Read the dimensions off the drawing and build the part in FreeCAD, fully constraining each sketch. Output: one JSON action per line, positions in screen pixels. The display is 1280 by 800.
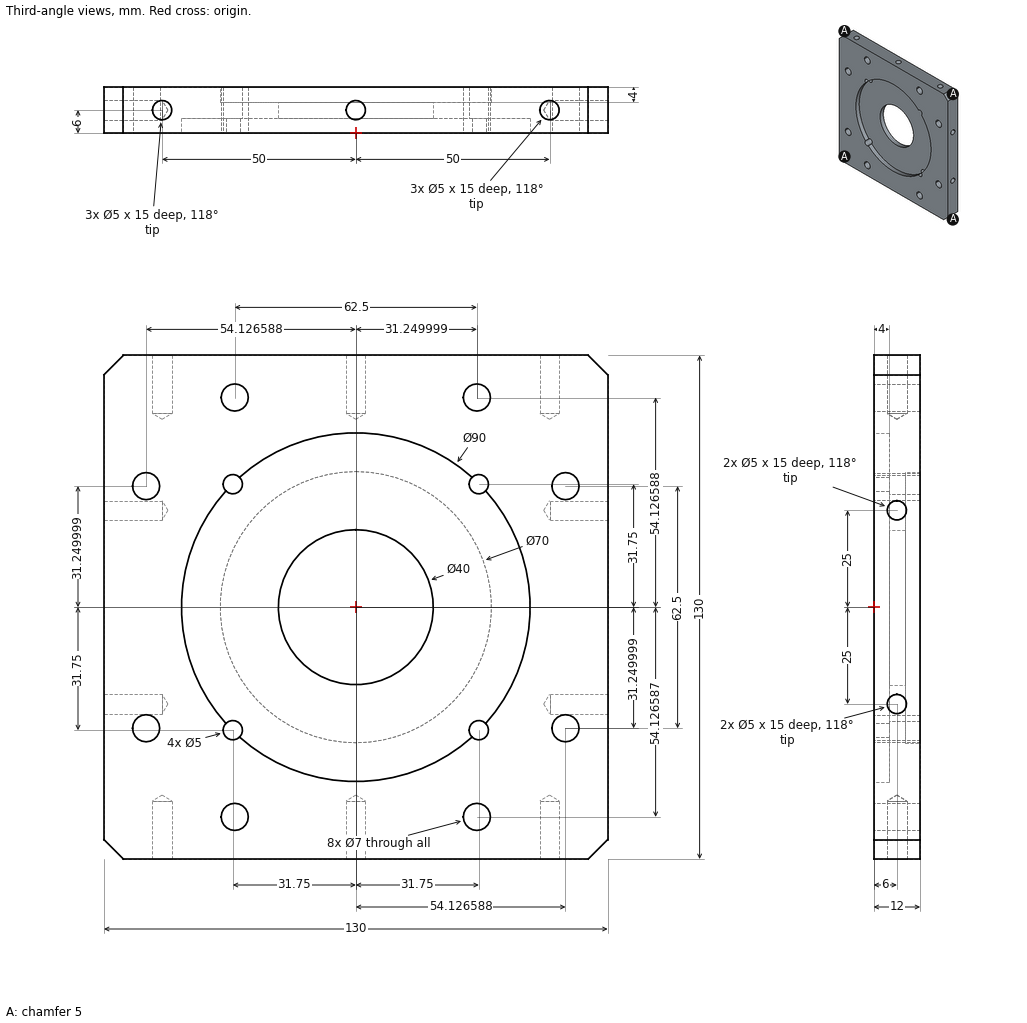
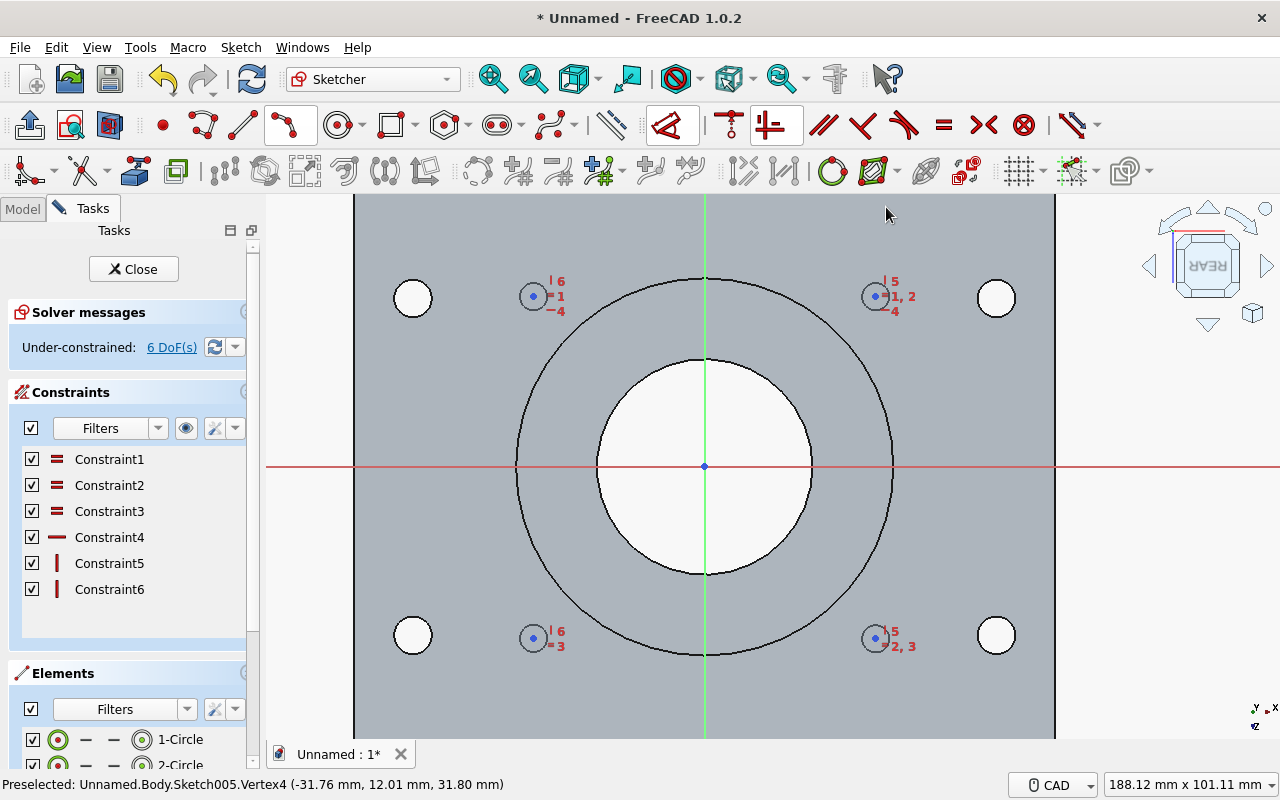
{"action": "left_click", "coordinate": [876, 639]}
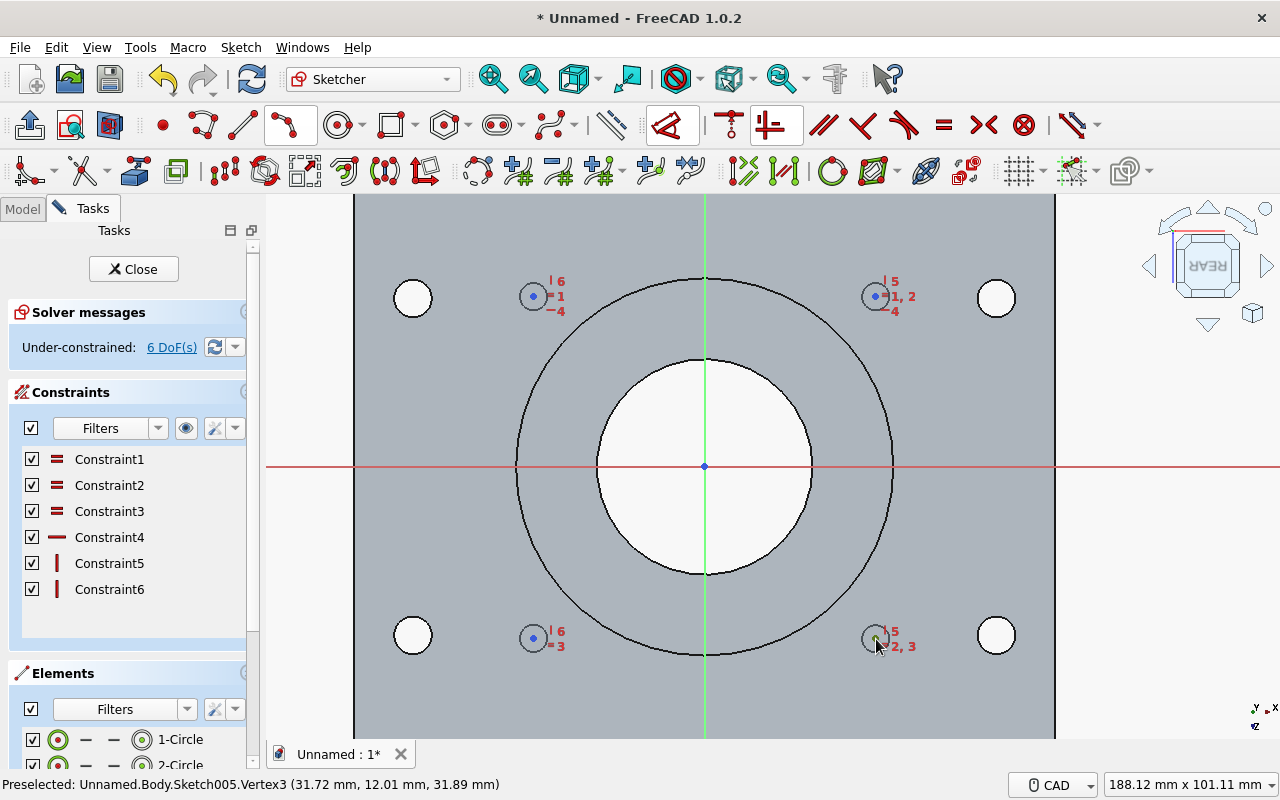
{"action": "left_click", "coordinate": [534, 638]}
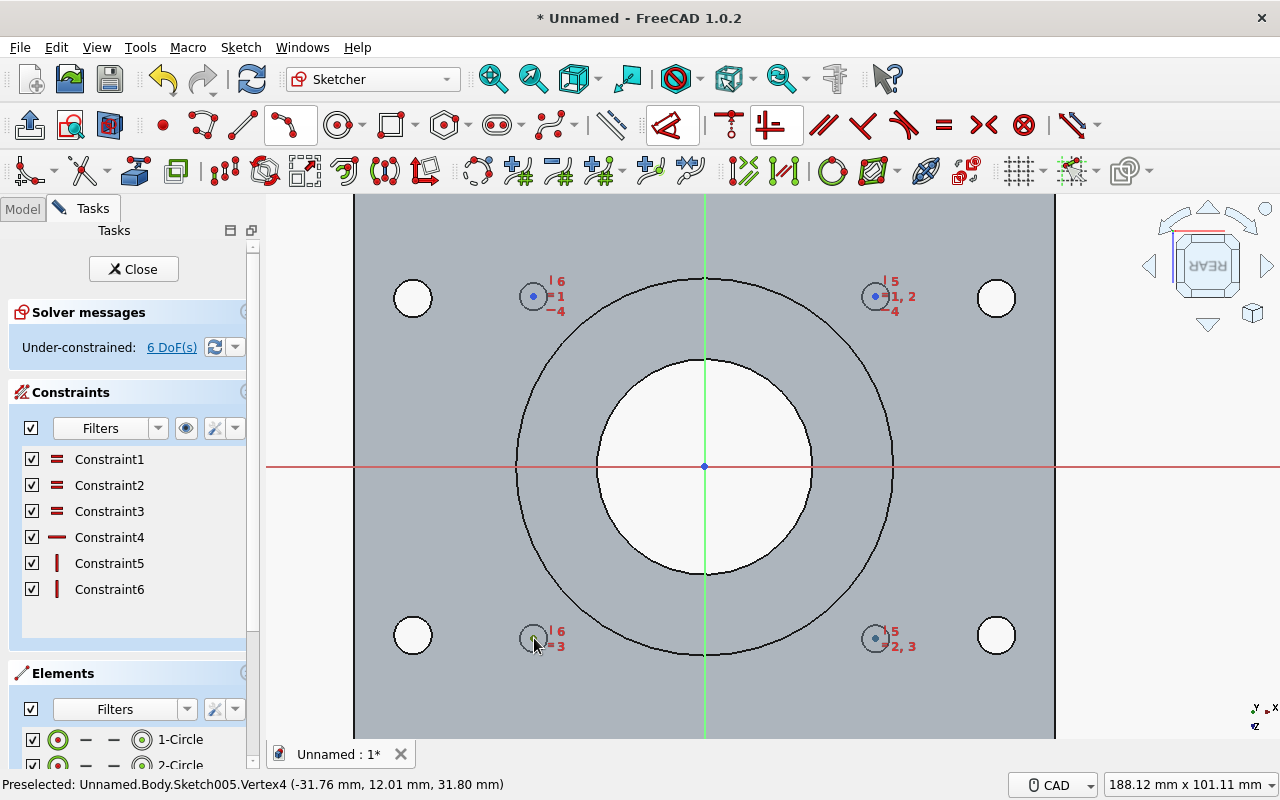
{"action": "key", "text": "h"}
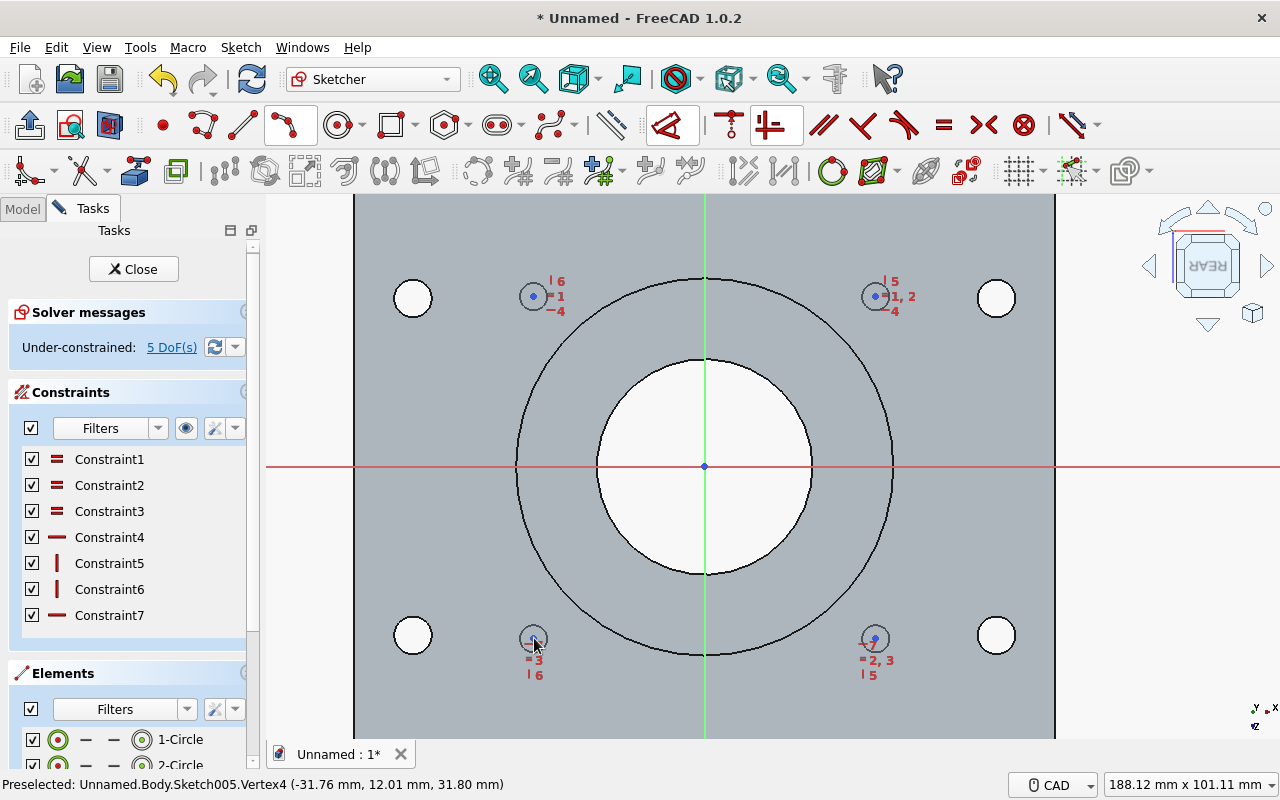
{"action": "key", "text": "d"}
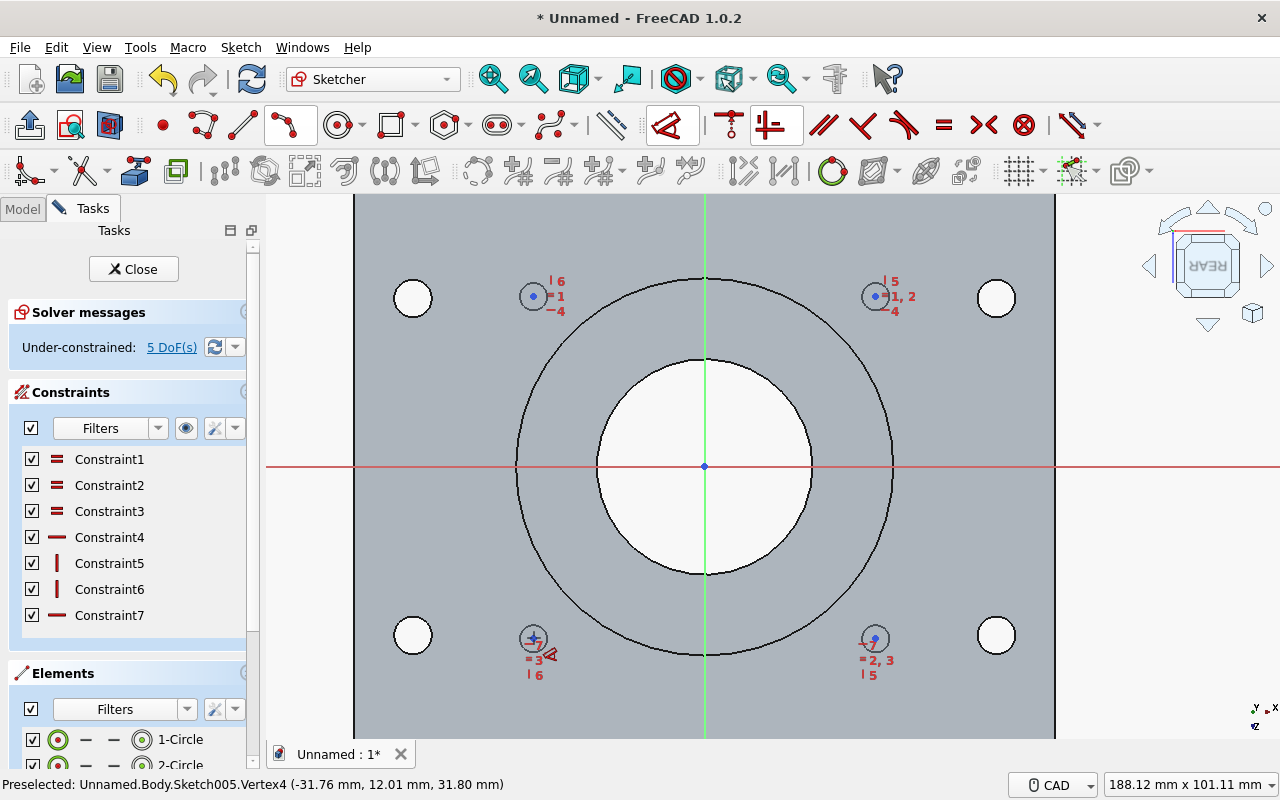
{"action": "scroll", "coordinate": [543, 287], "scroll_direction": "up", "scroll_amount": 2}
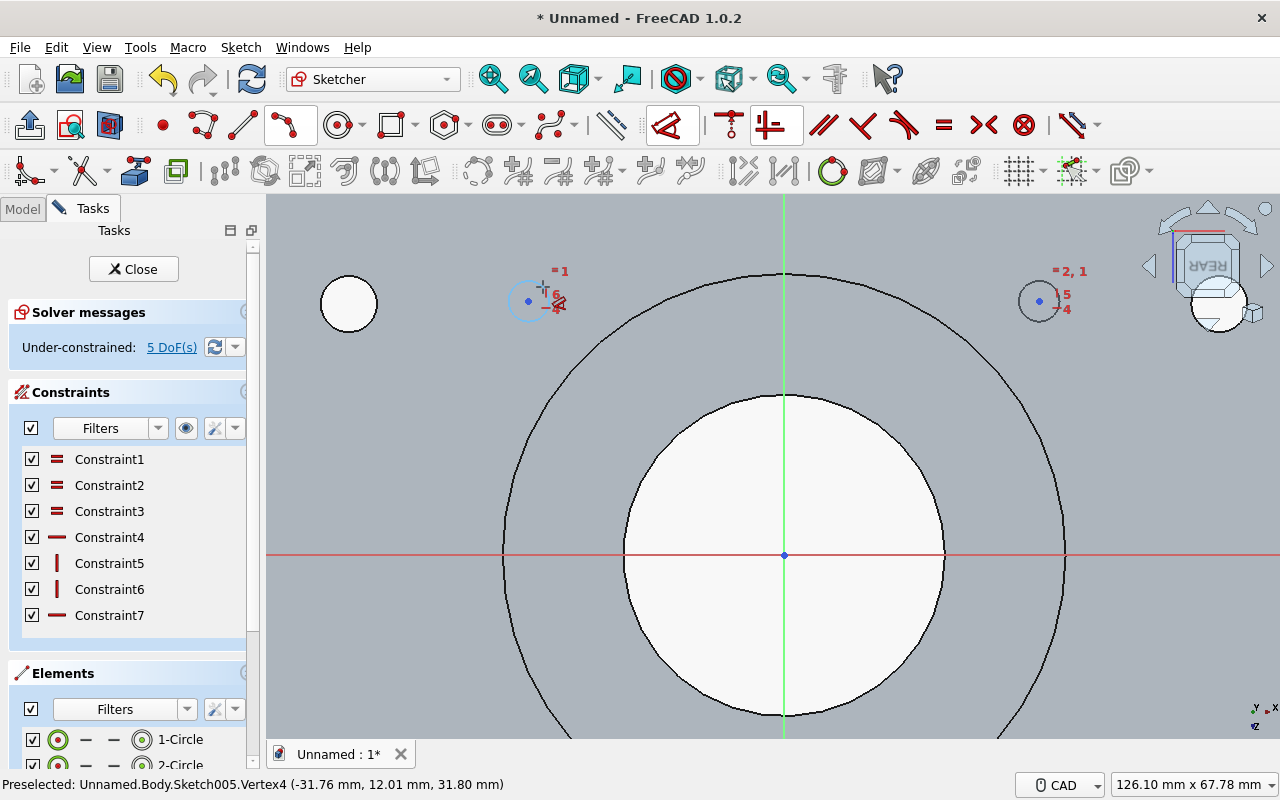
{"action": "left_click", "coordinate": [543, 287]}
{"action": "left_click", "coordinate": [566, 264]}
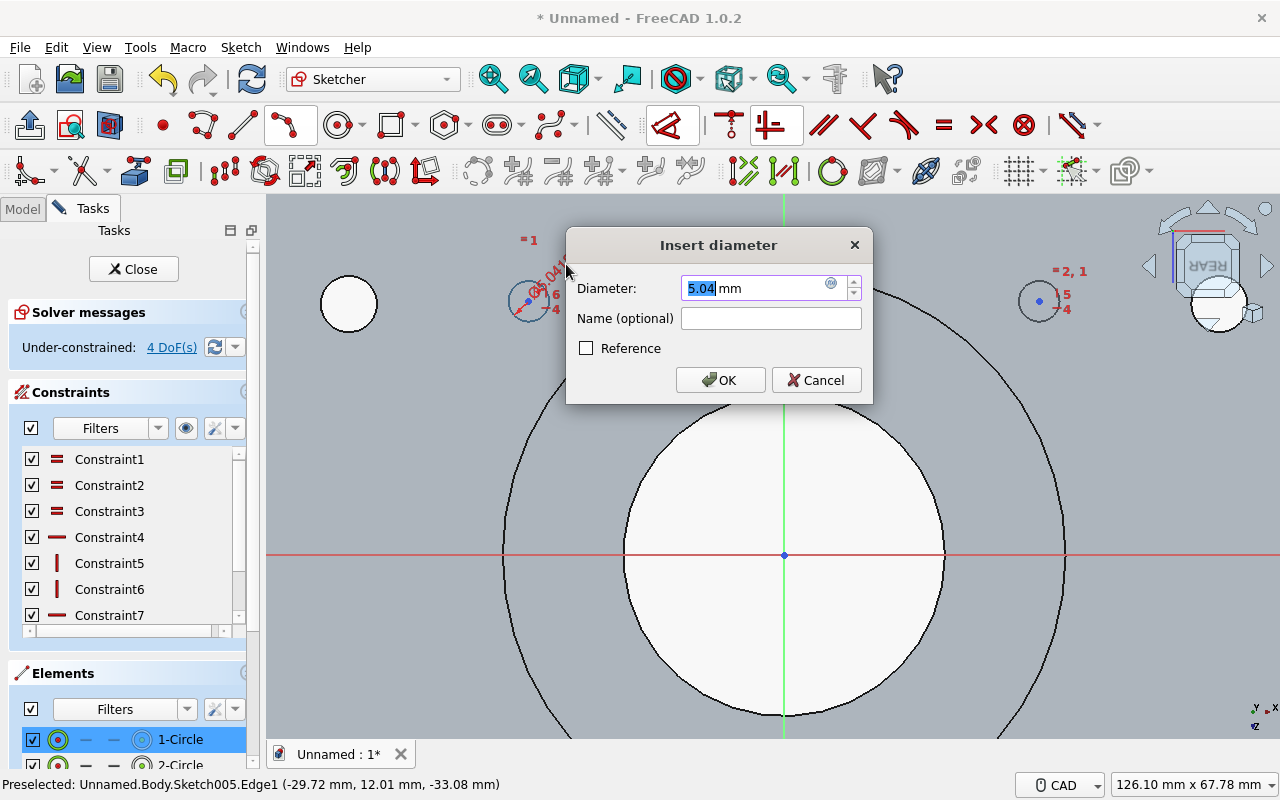
{"action": "type", "text": "5"}
{"action": "key", "text": "Return"}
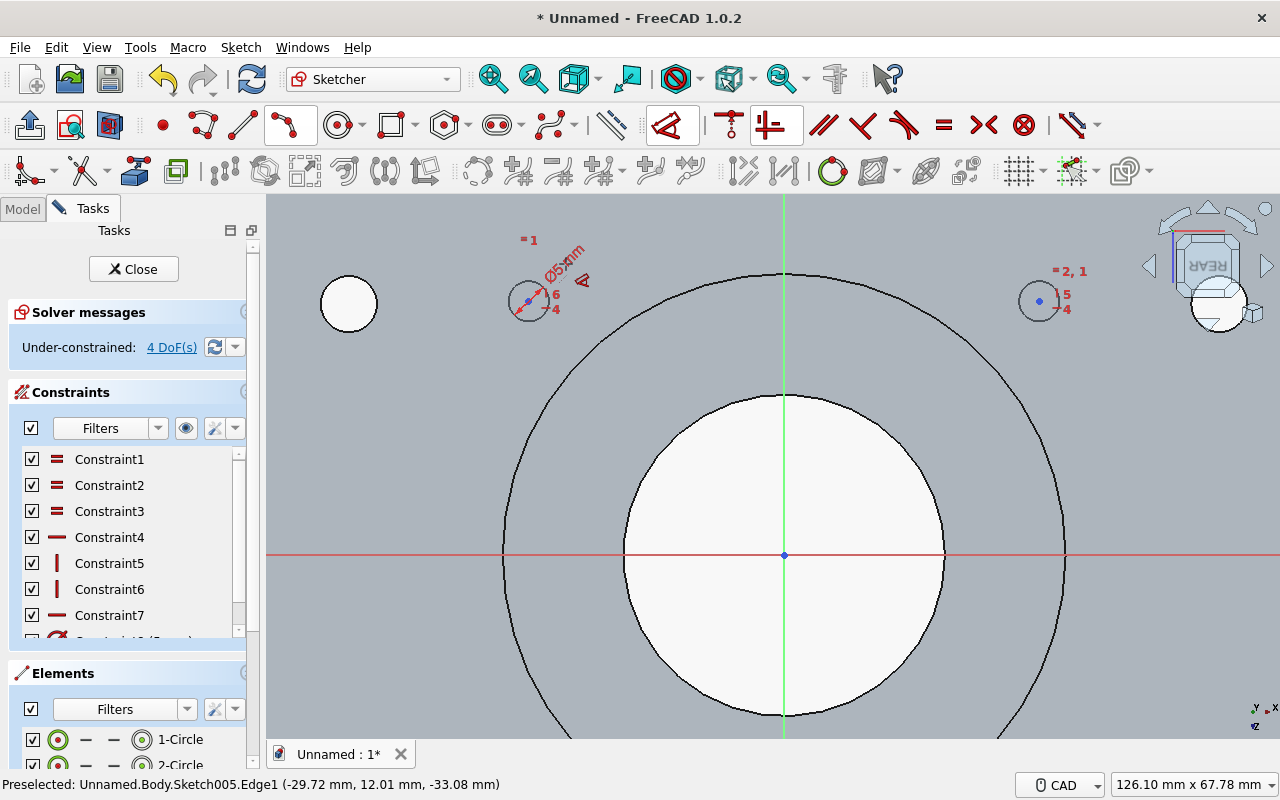
{"action": "left_click", "coordinate": [529, 301]}
{"action": "left_click", "coordinate": [656, 267]}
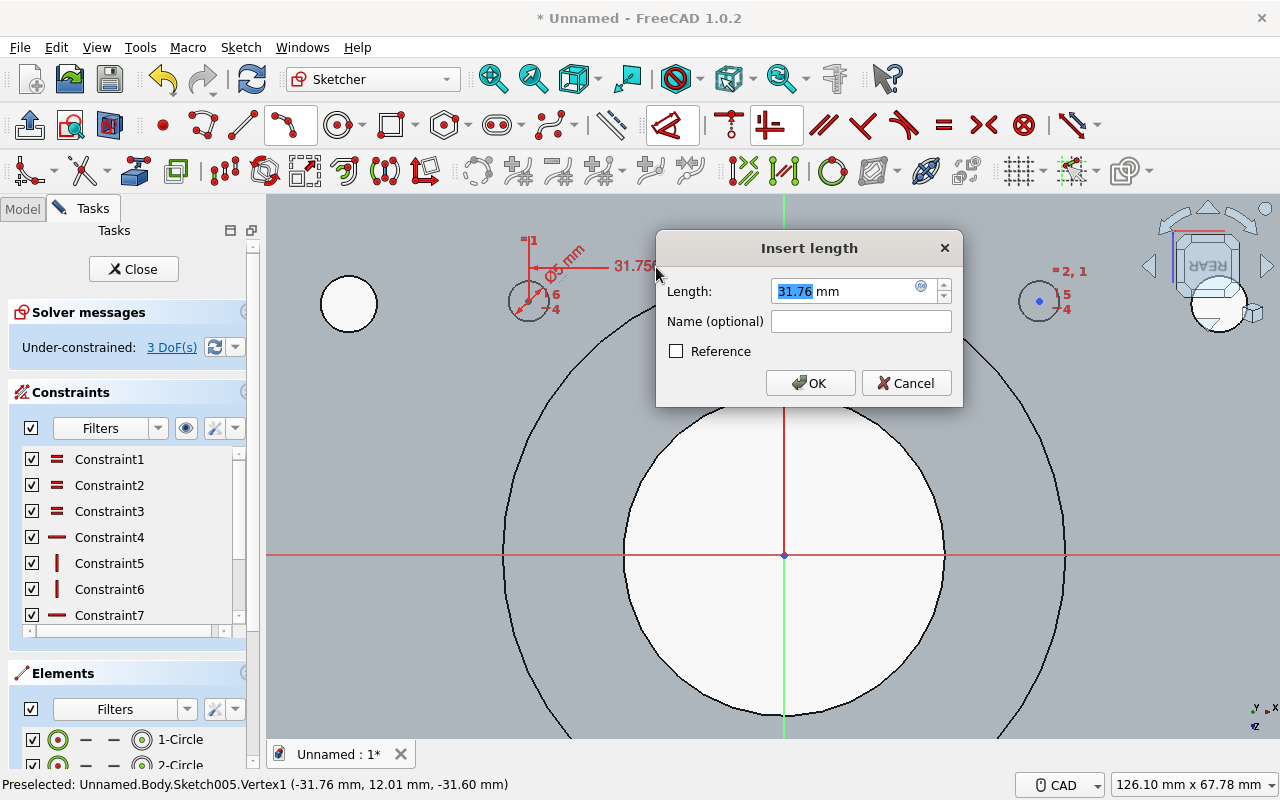
{"action": "type", "text": "31.75"}
{"action": "key", "text": "Return"}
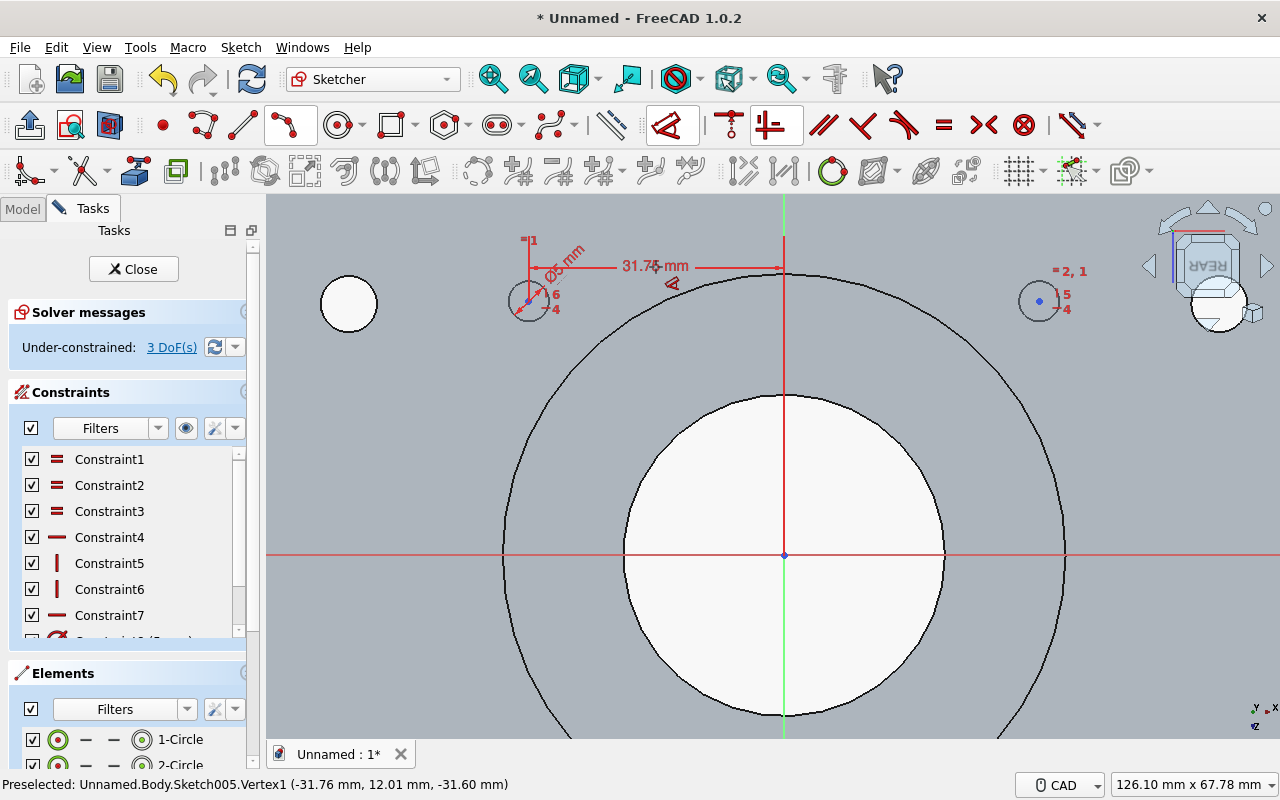
{"action": "left_click", "coordinate": [529, 301]}
{"action": "left_click", "coordinate": [495, 428]}